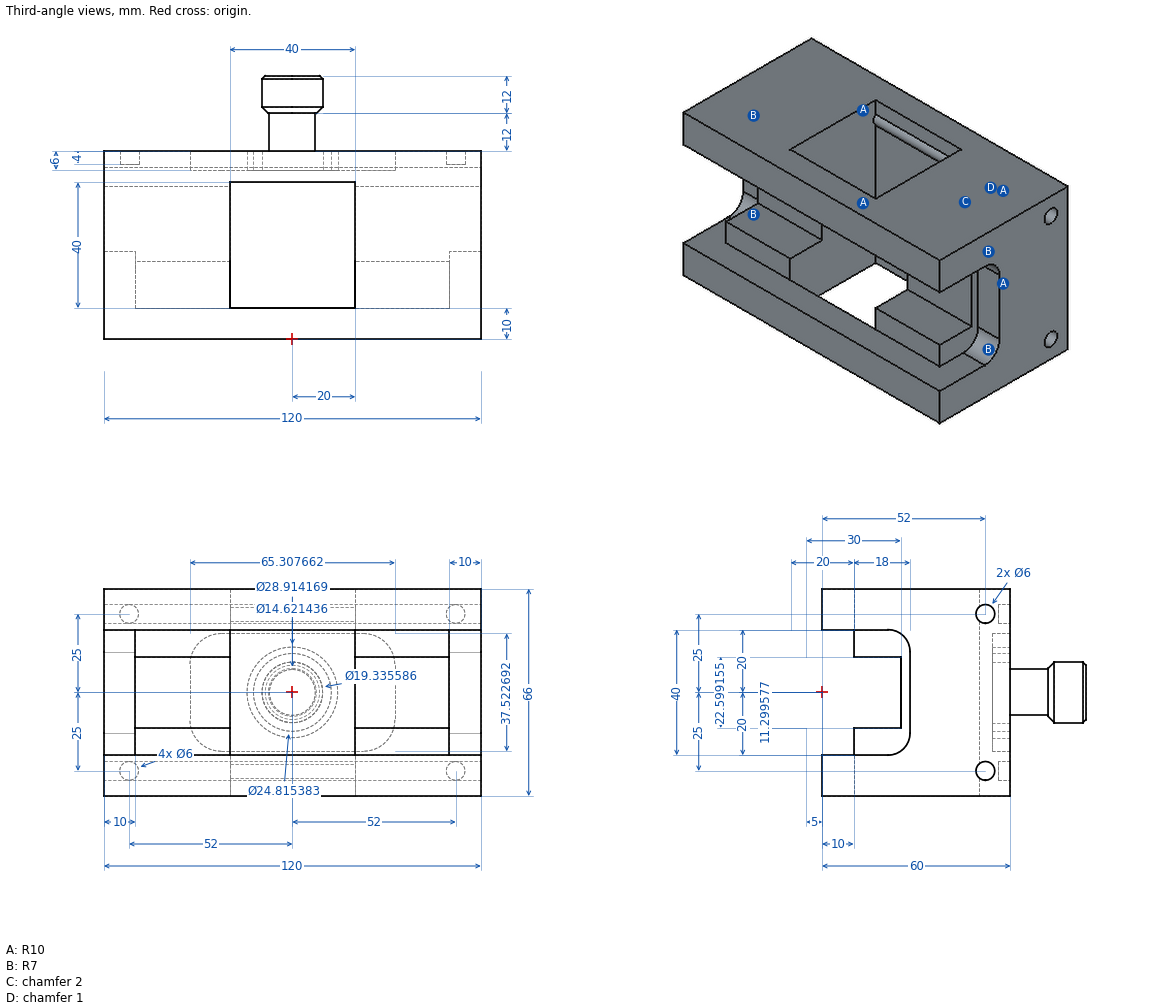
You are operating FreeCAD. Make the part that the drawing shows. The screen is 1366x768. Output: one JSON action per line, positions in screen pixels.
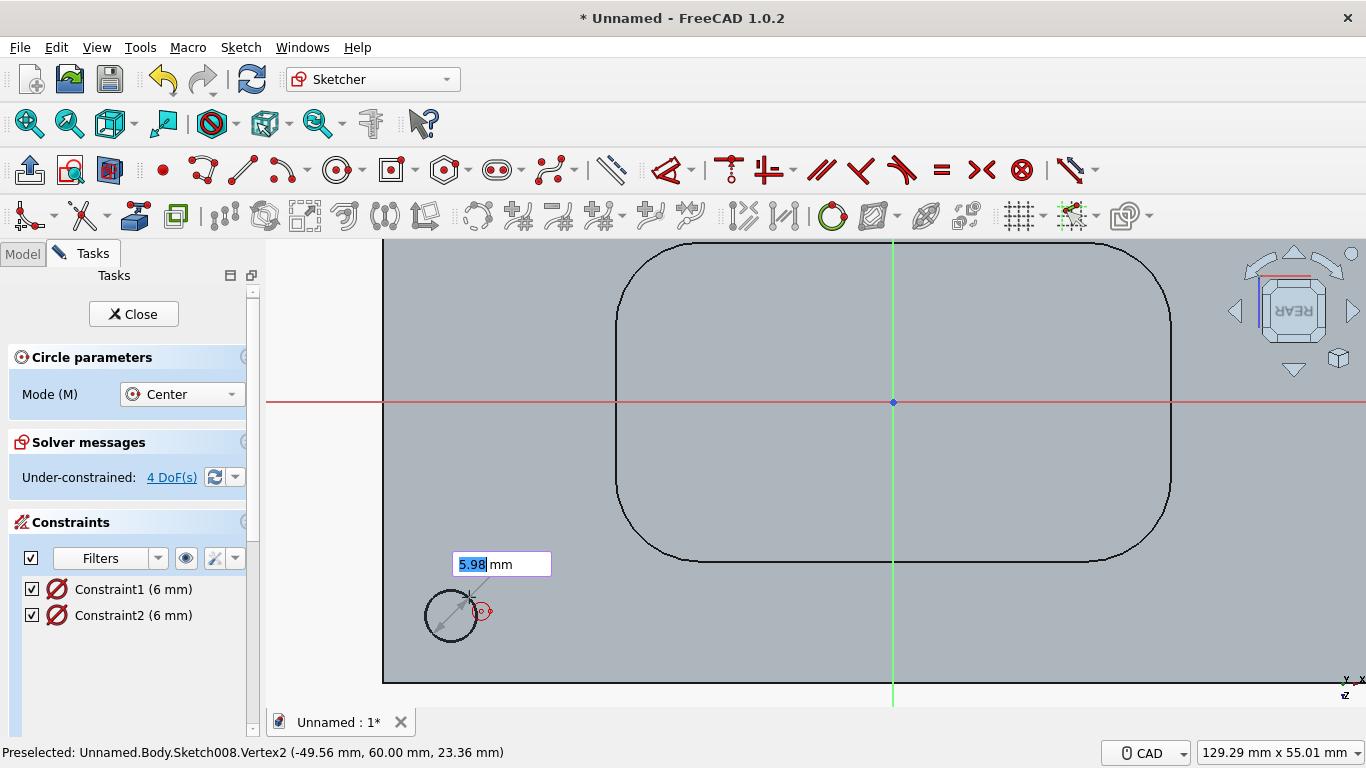
{"action": "type", "text": "6"}
{"action": "key", "text": "Return"}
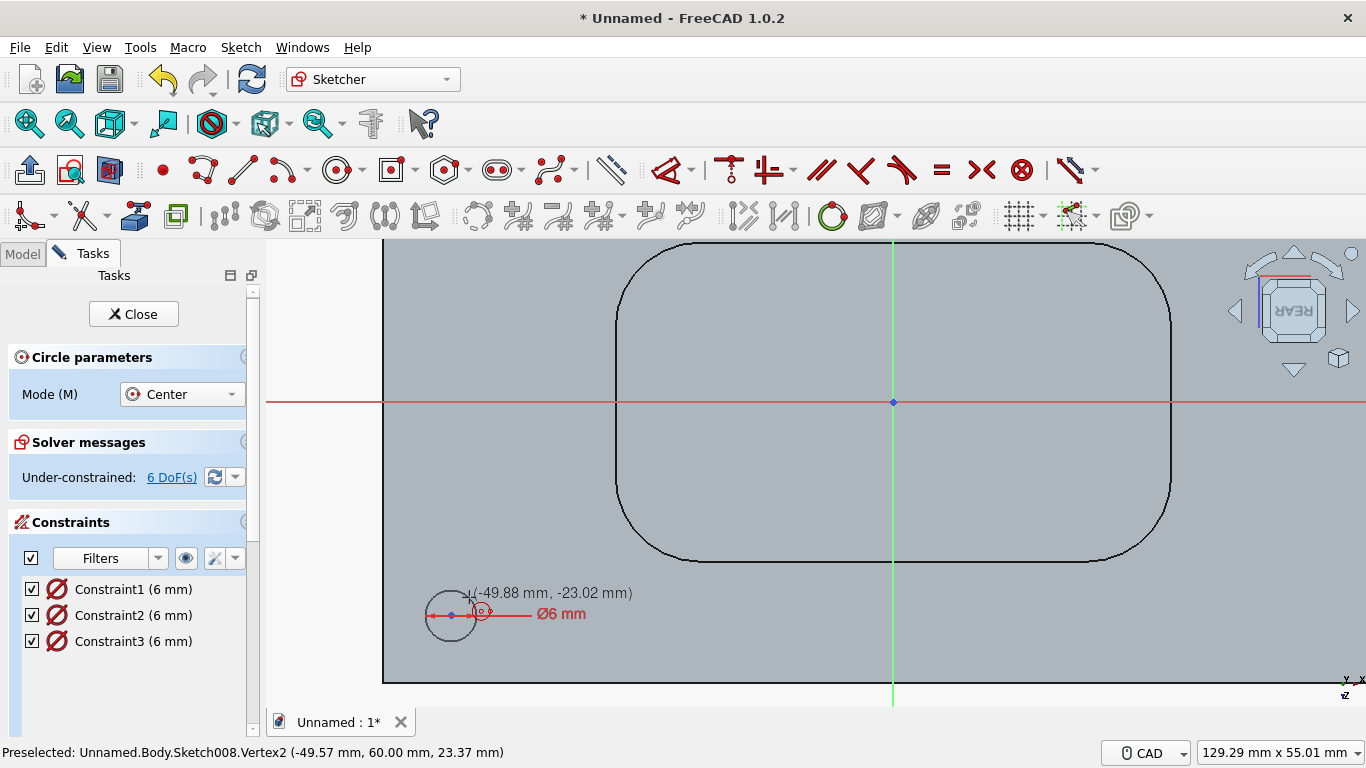
{"action": "scroll", "coordinate": [451, 617], "scroll_direction": "down", "scroll_amount": 2}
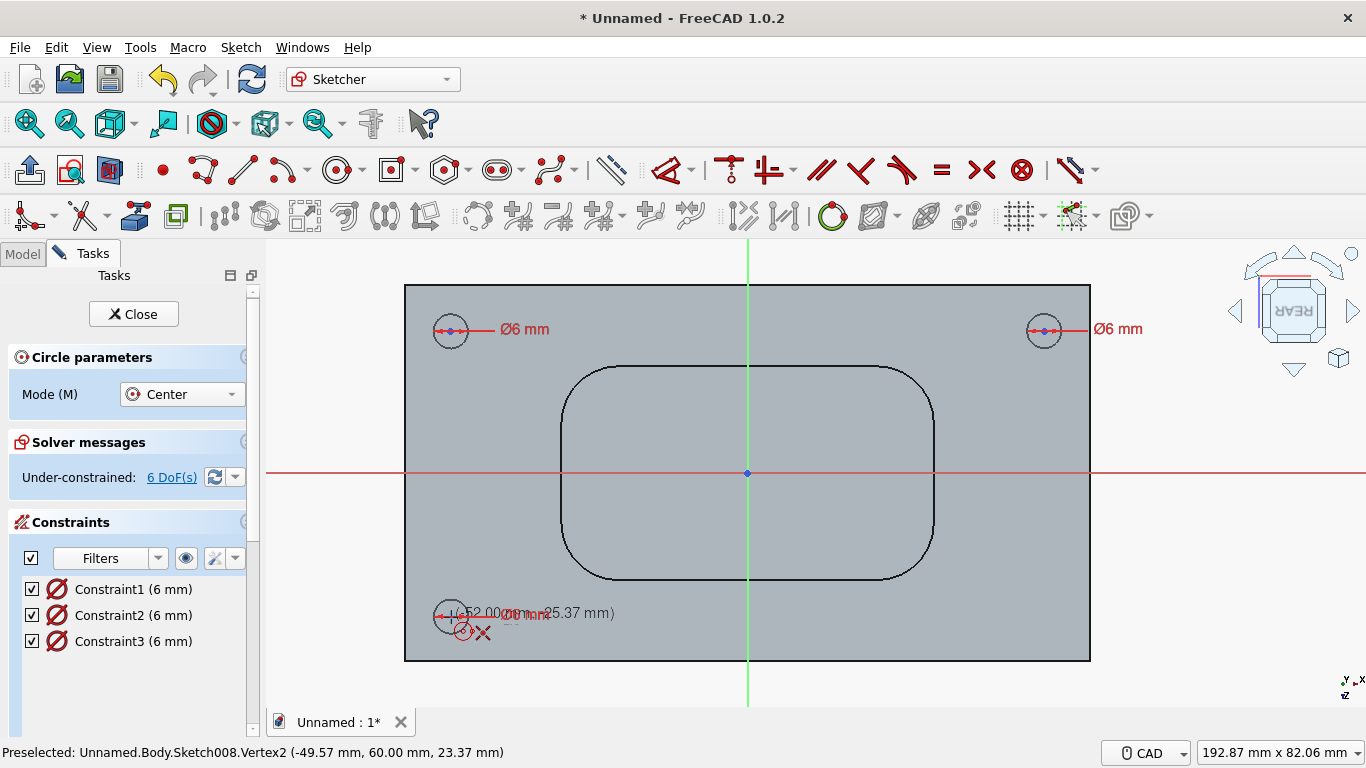
{"action": "scroll", "coordinate": [1044, 616], "scroll_direction": "up", "scroll_amount": 2}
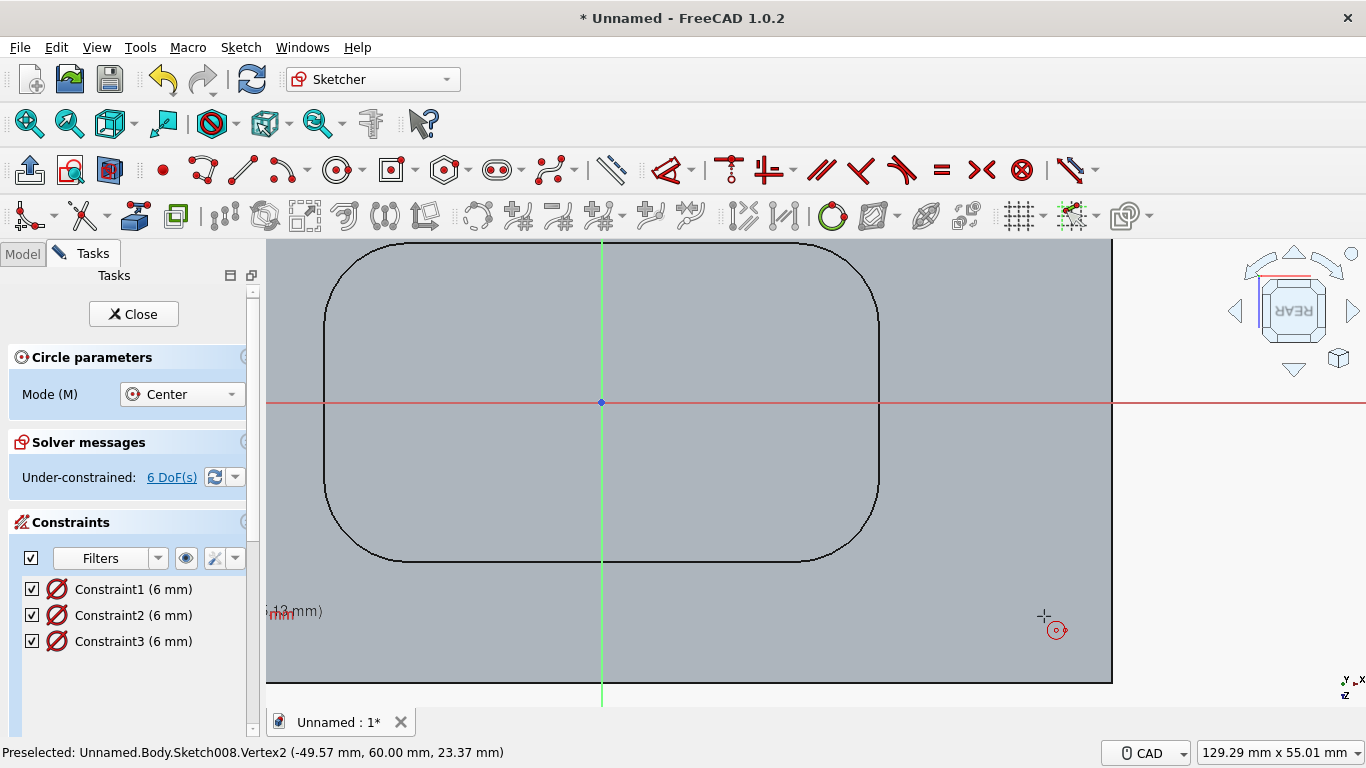
{"action": "left_click", "coordinate": [1044, 615]}
{"action": "mouse_move", "coordinate": [1062, 597]}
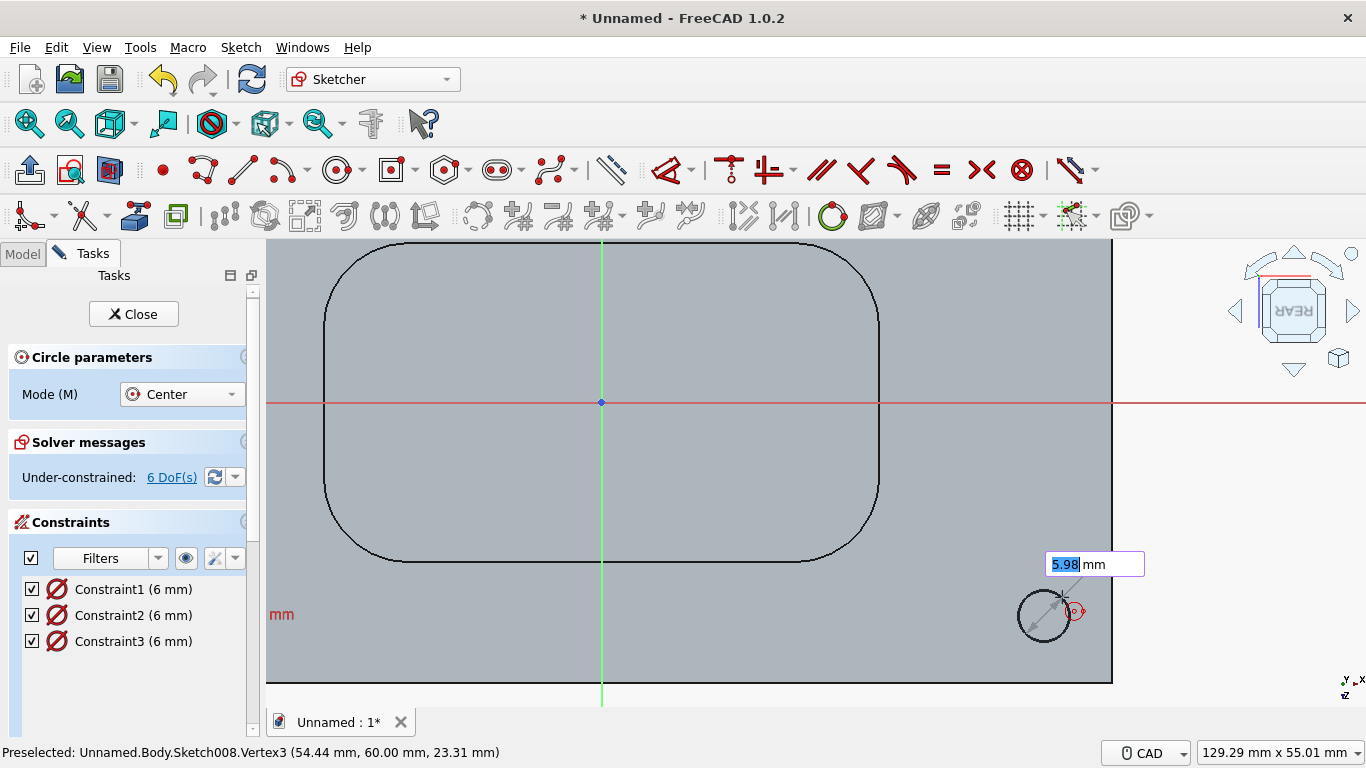
{"action": "type", "text": "6"}
{"action": "key", "text": "Return"}
{"action": "key", "text": "Escape"}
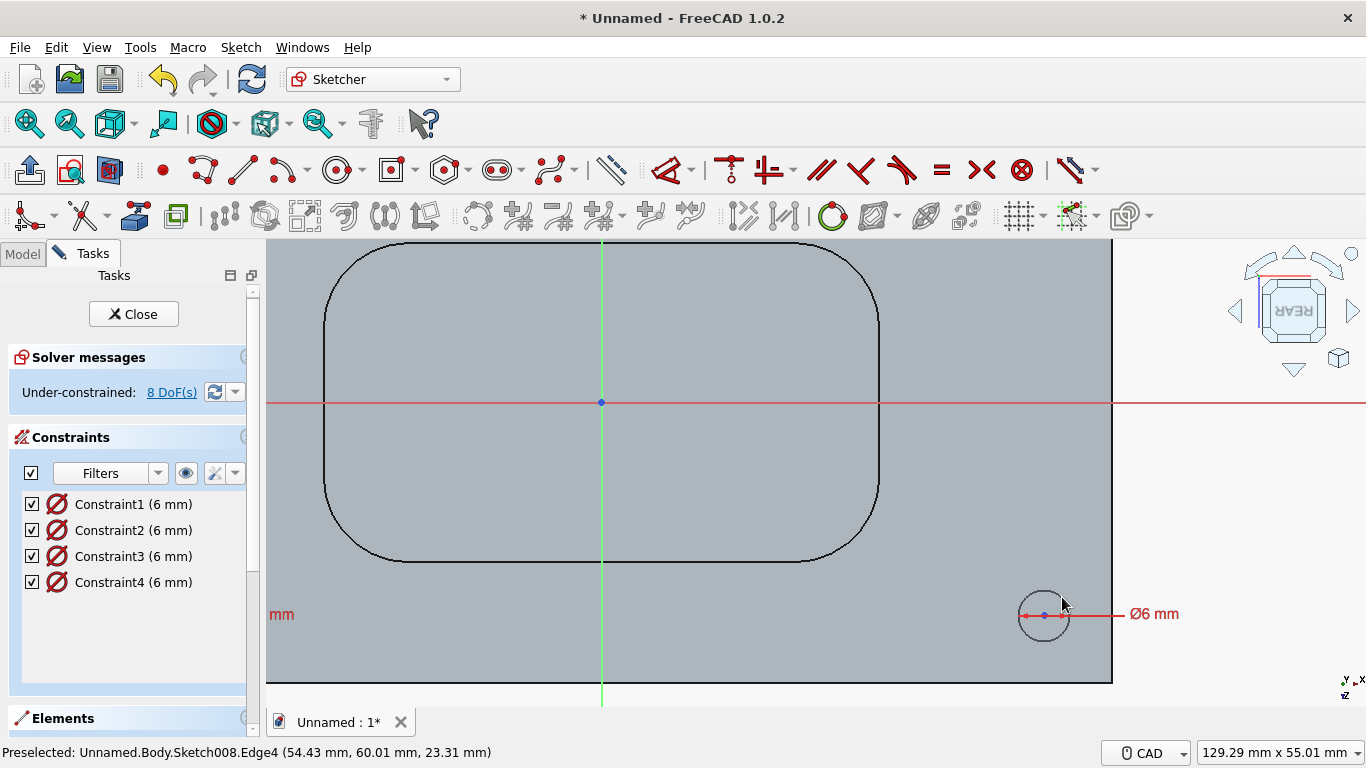
{"action": "scroll", "coordinate": [1044, 616], "scroll_direction": "down", "scroll_amount": 2}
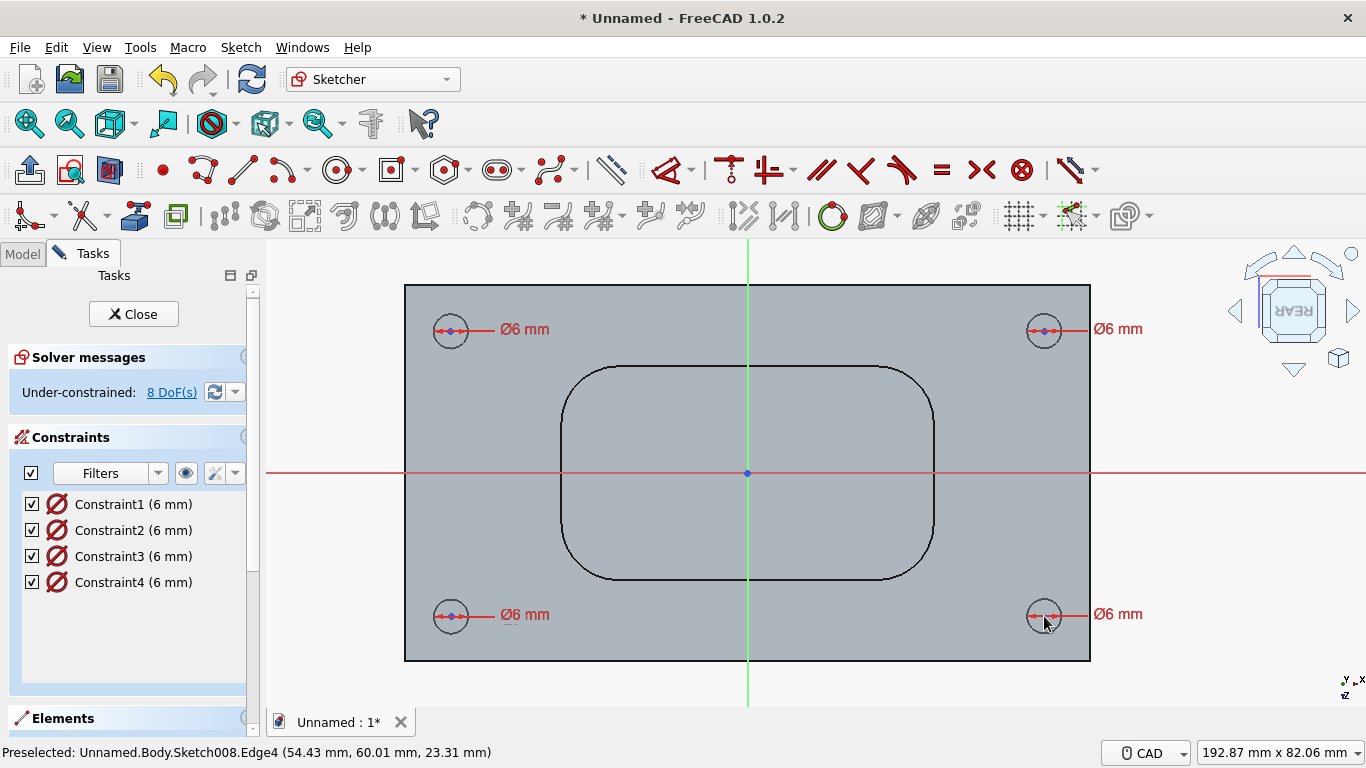
{"action": "left_click", "coordinate": [451, 331]}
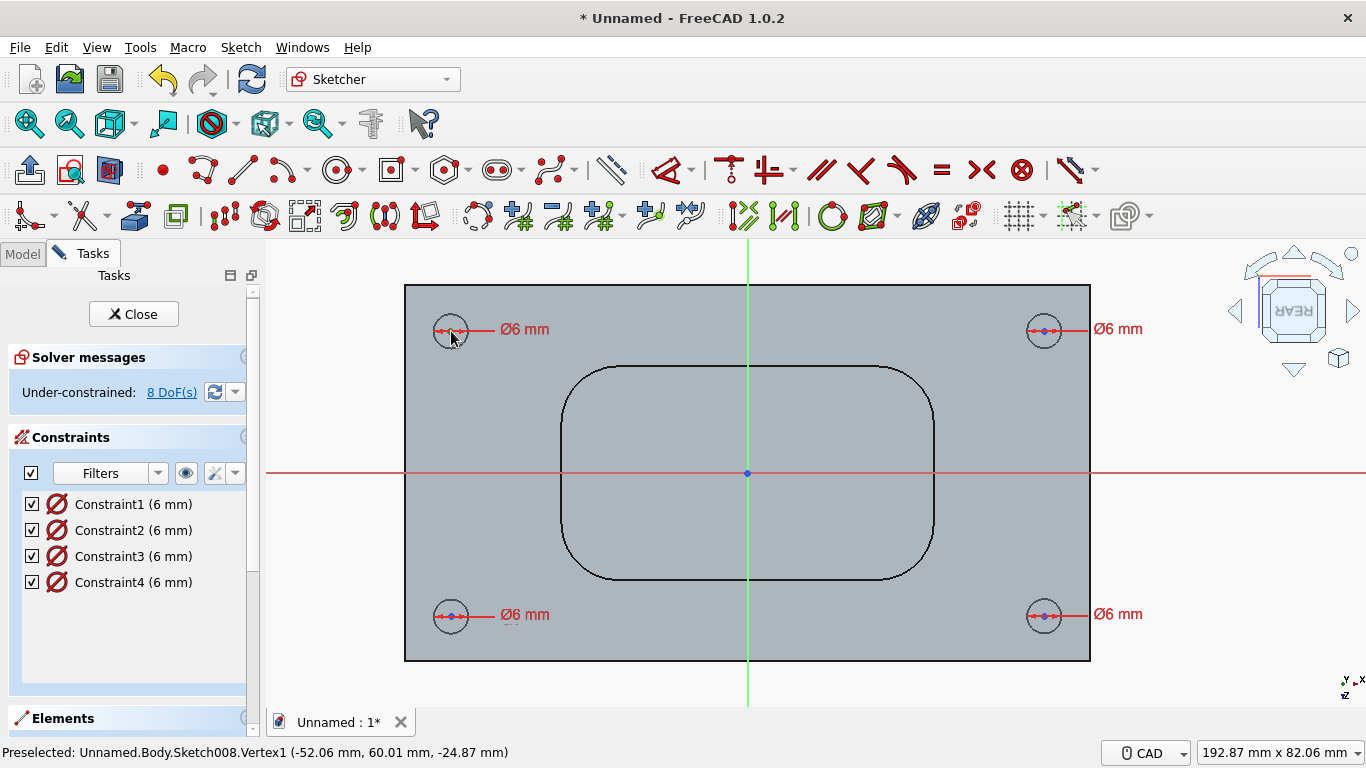
{"action": "left_click", "coordinate": [1044, 331]}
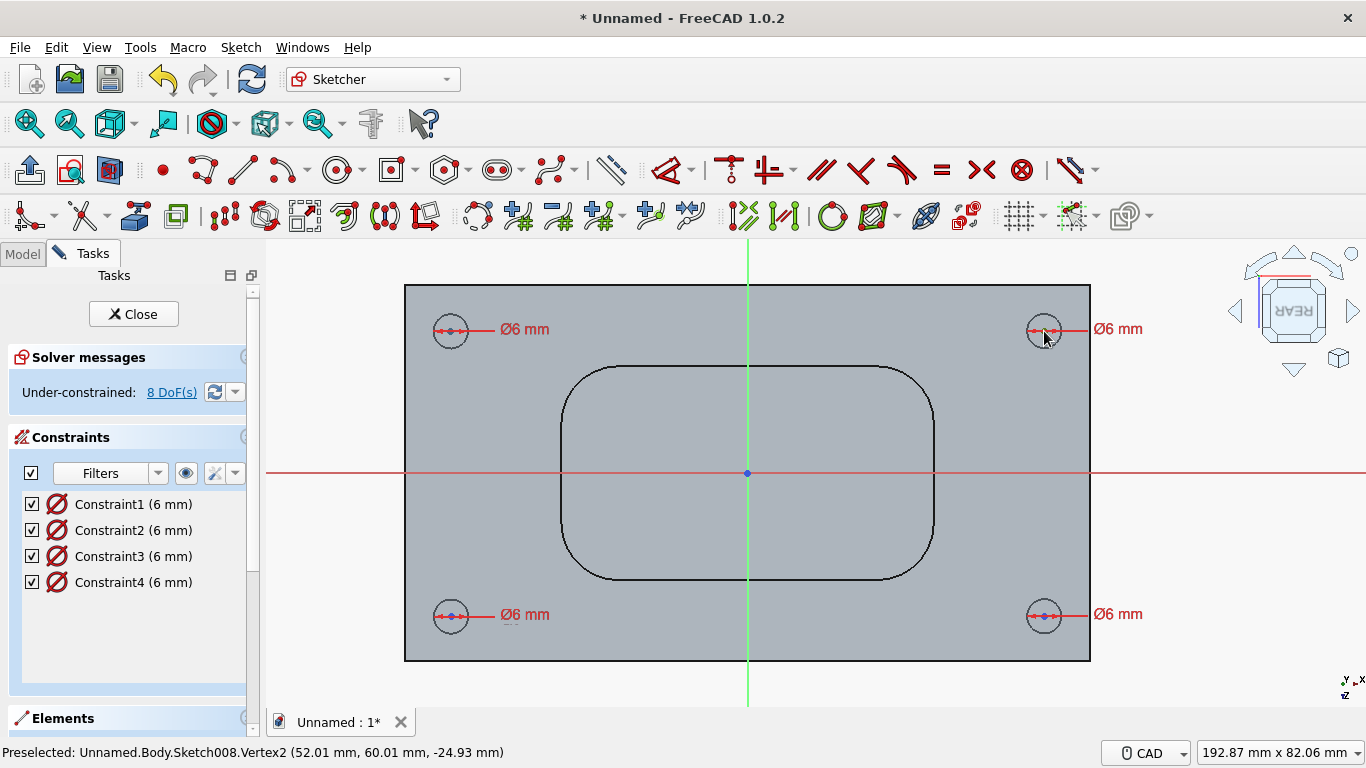
{"action": "left_click", "coordinate": [796, 170]}